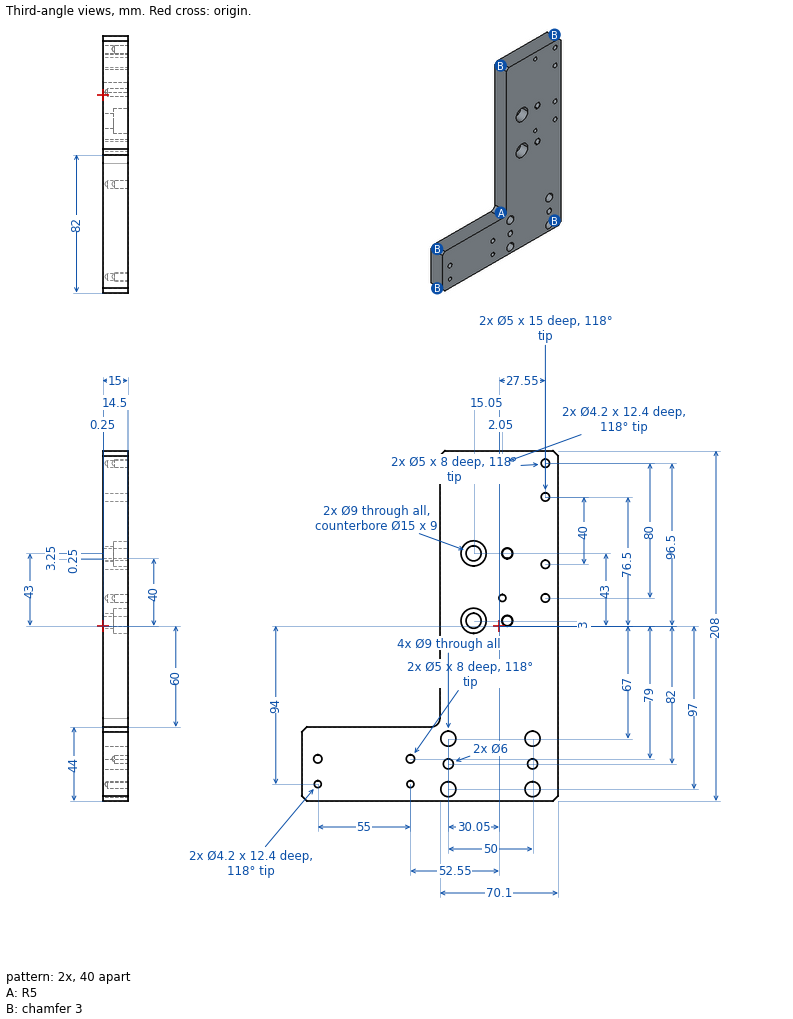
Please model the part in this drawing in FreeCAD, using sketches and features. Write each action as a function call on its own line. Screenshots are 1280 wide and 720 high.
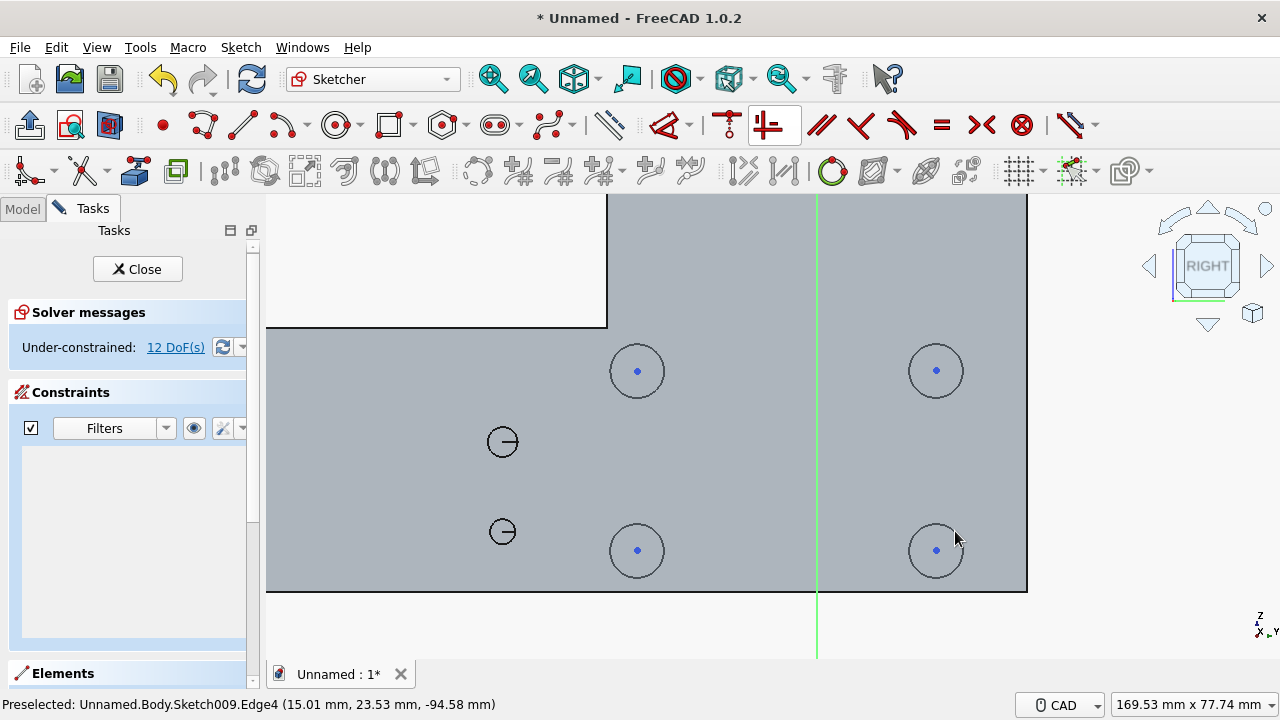
click(656, 352)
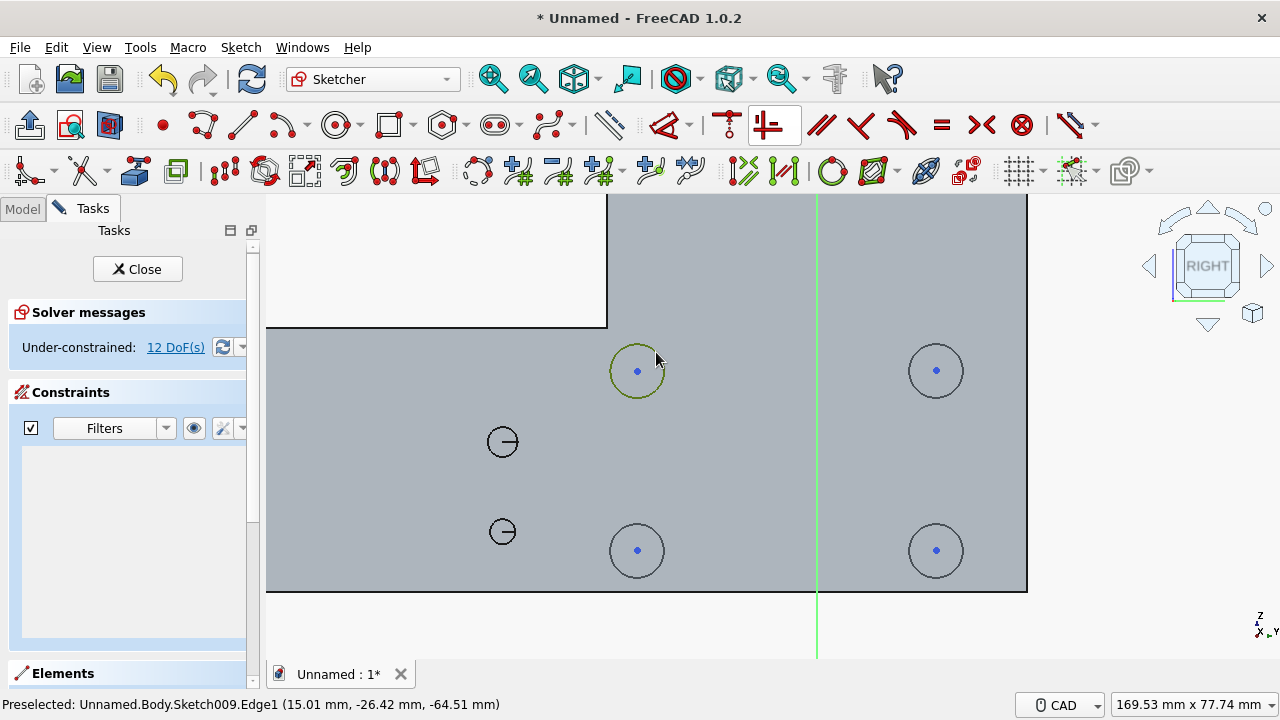
click(656, 532)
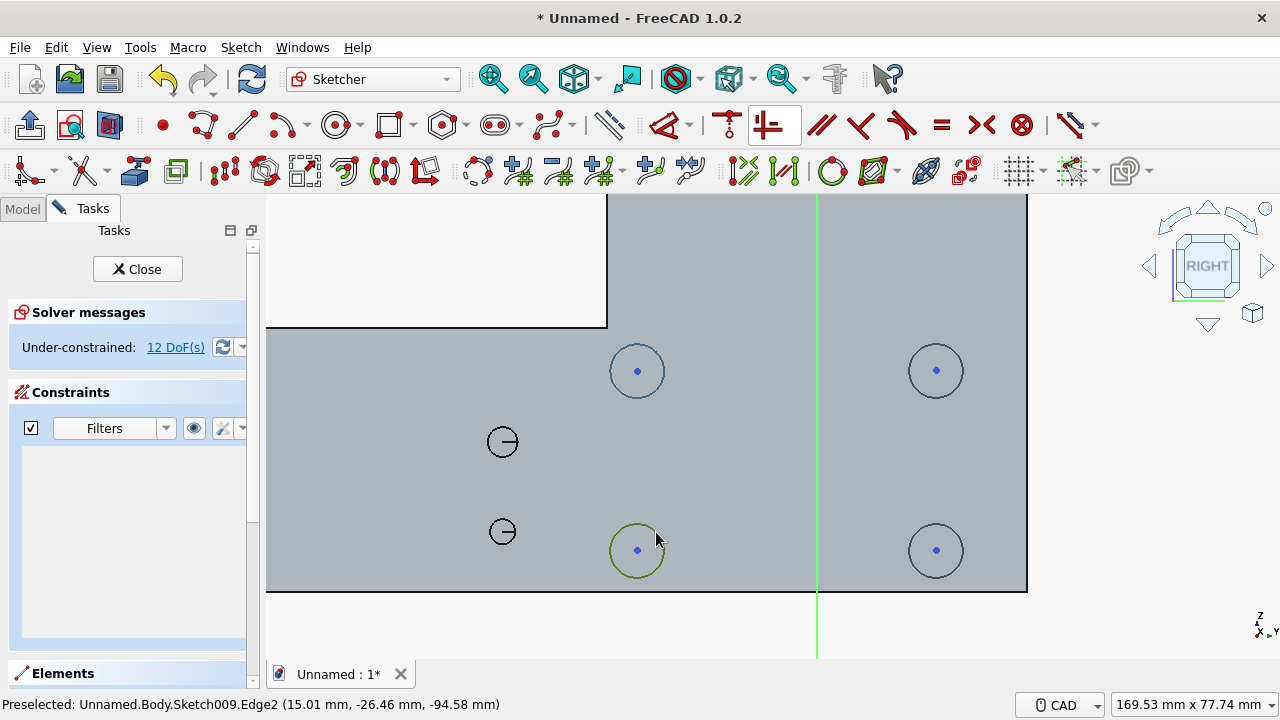
click(955, 352)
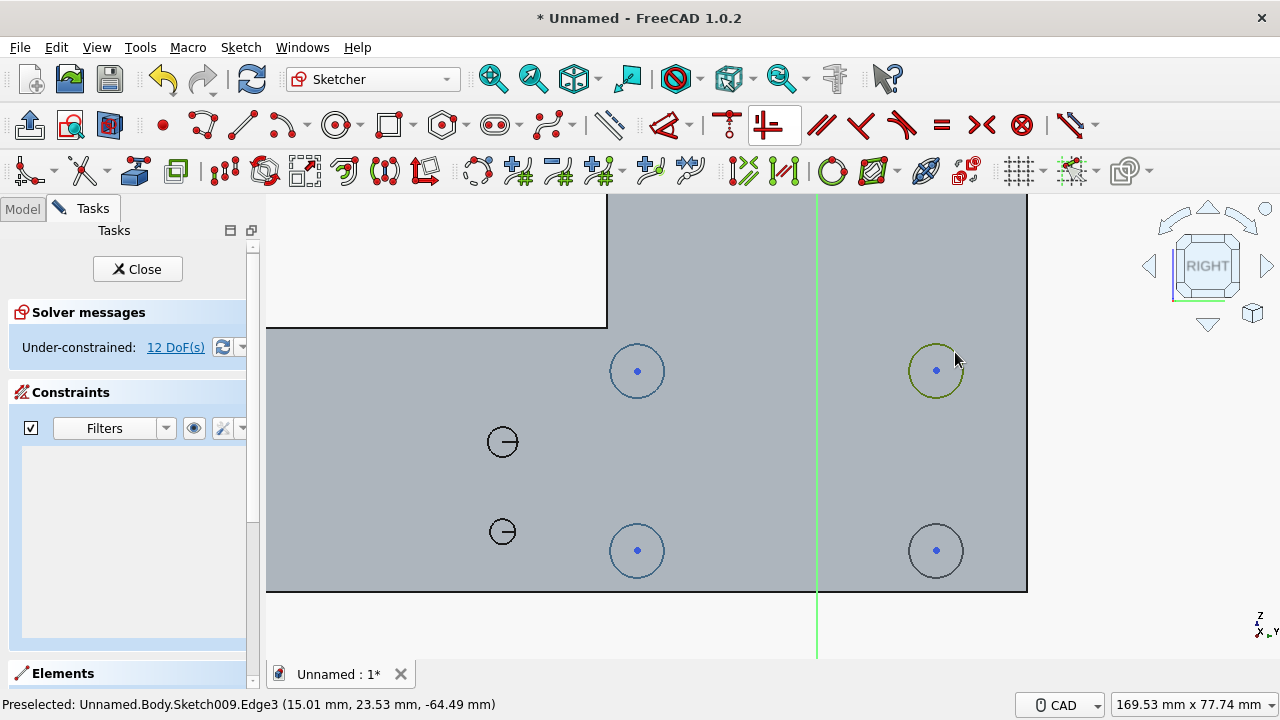
click(955, 532)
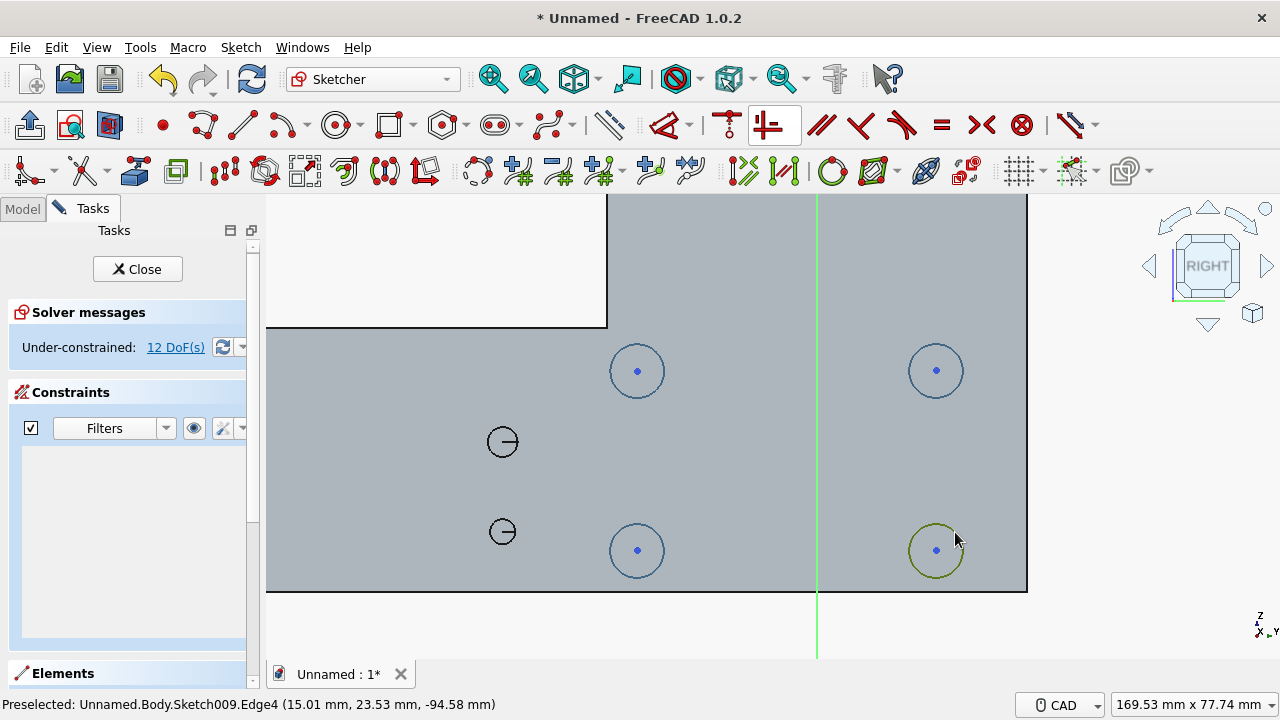
key(e)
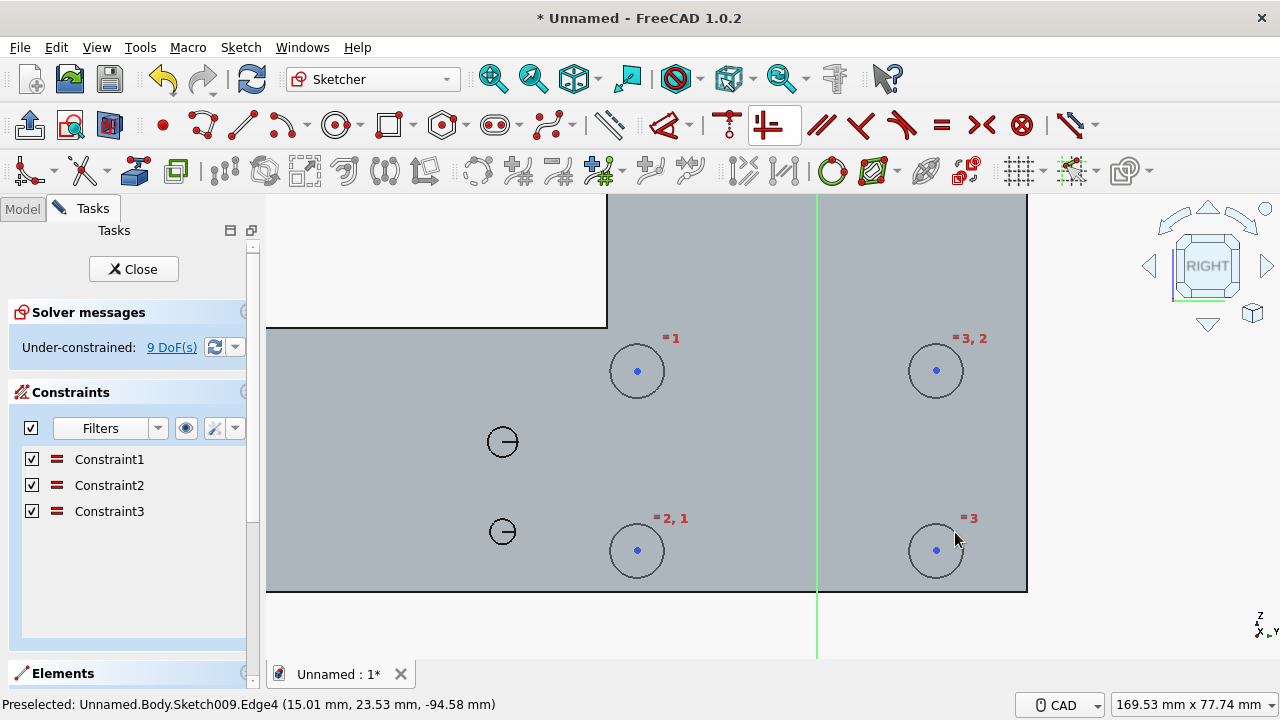
click(637, 371)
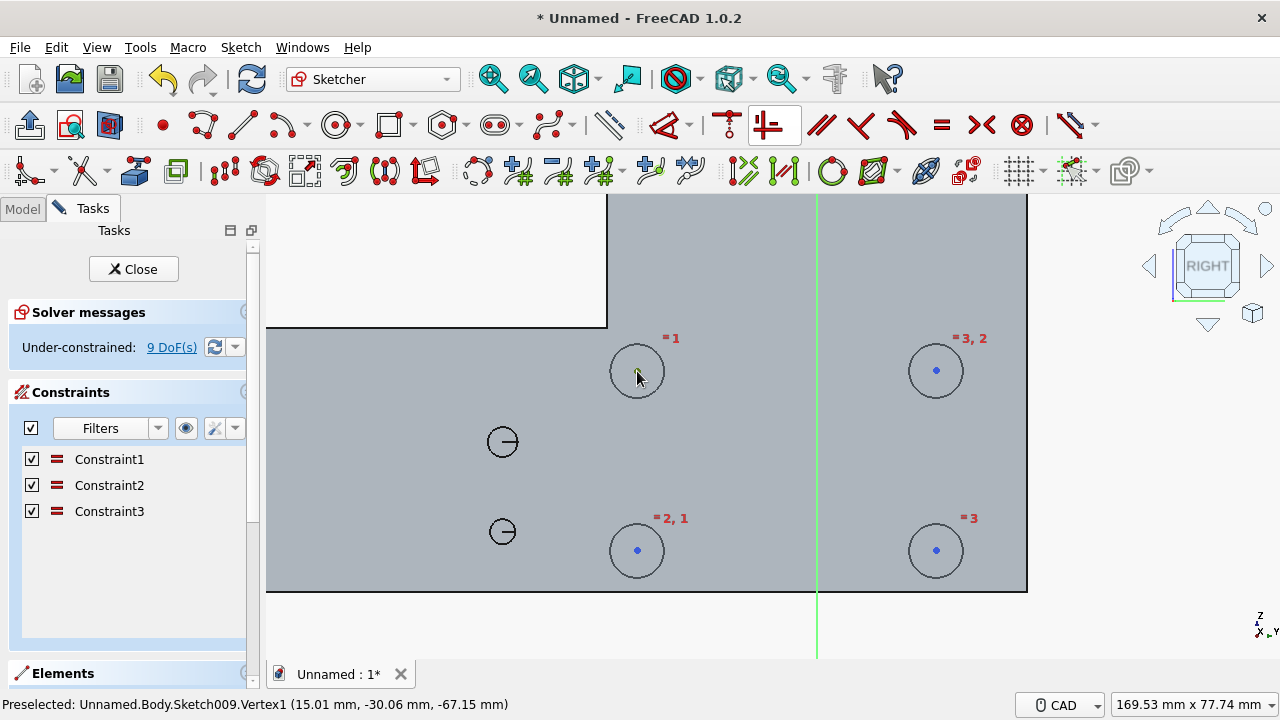
click(637, 551)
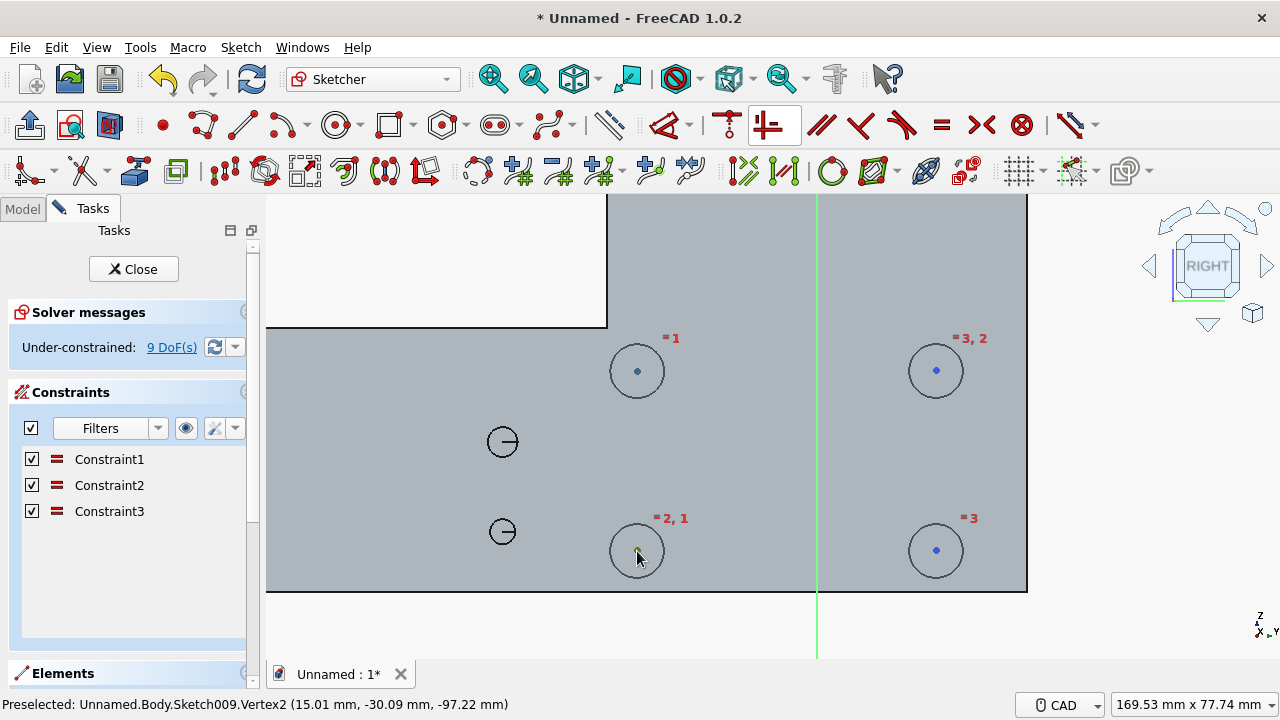
key(v)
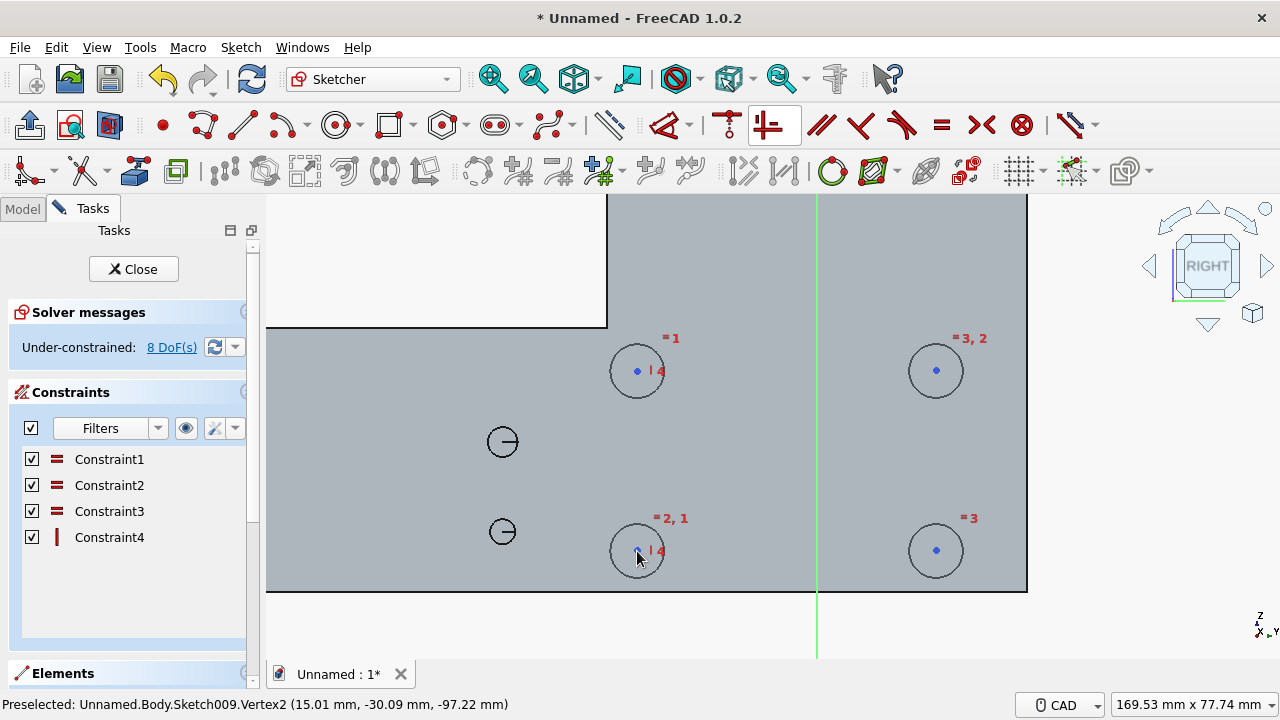
click(637, 371)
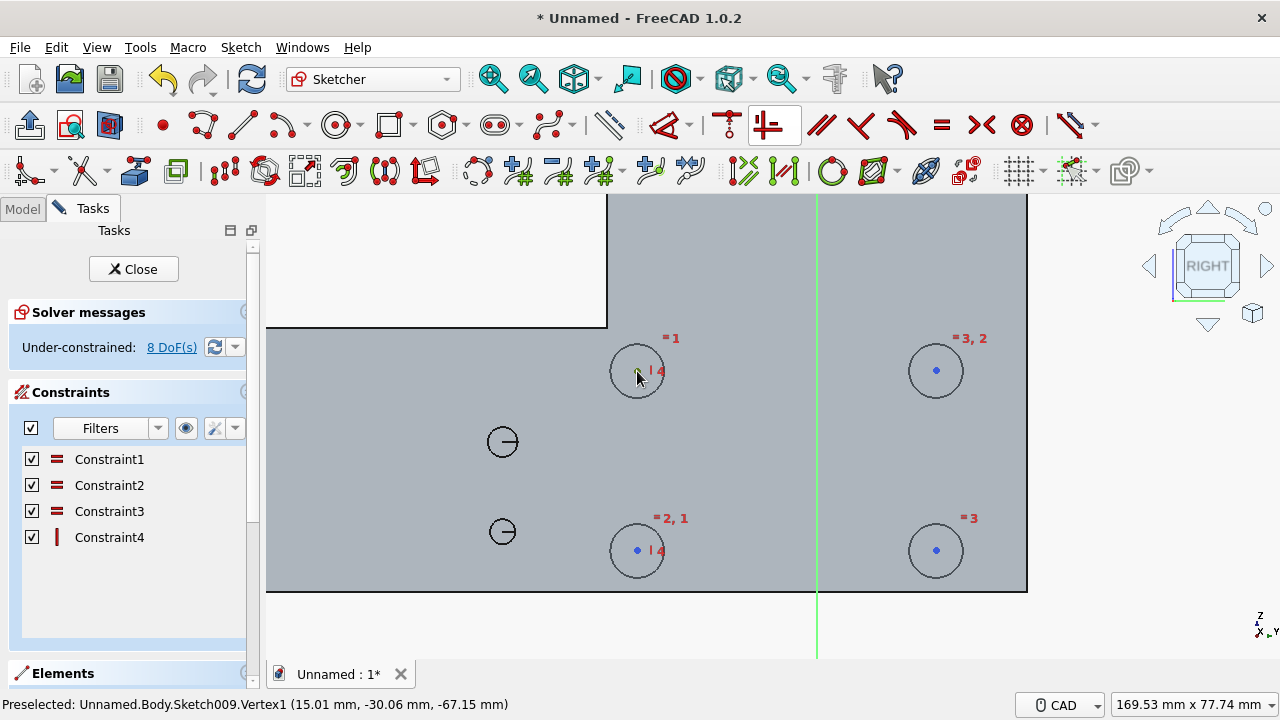
click(936, 371)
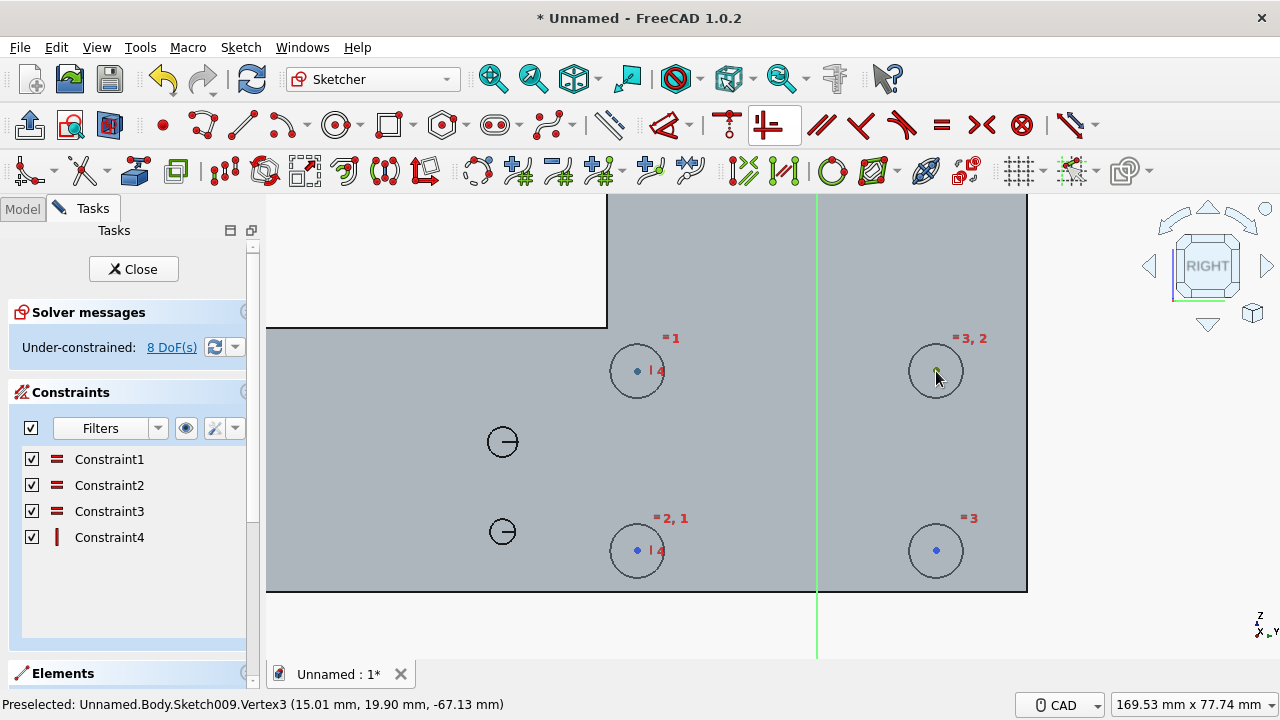
click(796, 126)